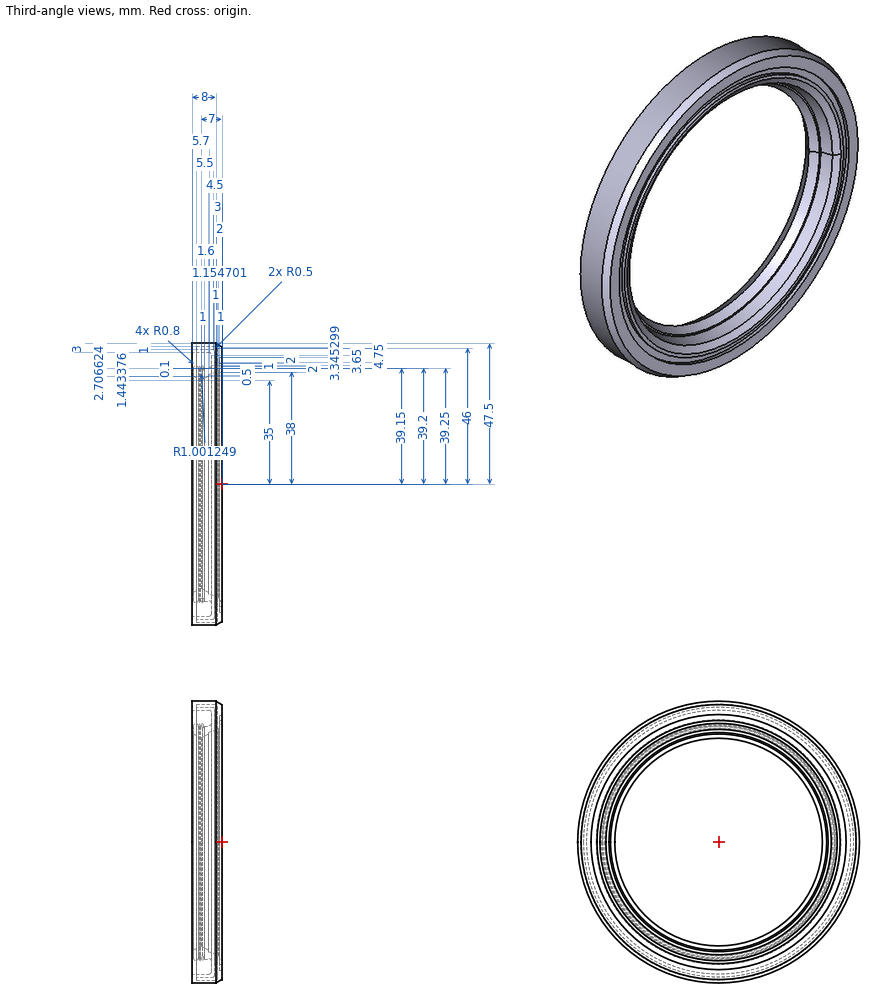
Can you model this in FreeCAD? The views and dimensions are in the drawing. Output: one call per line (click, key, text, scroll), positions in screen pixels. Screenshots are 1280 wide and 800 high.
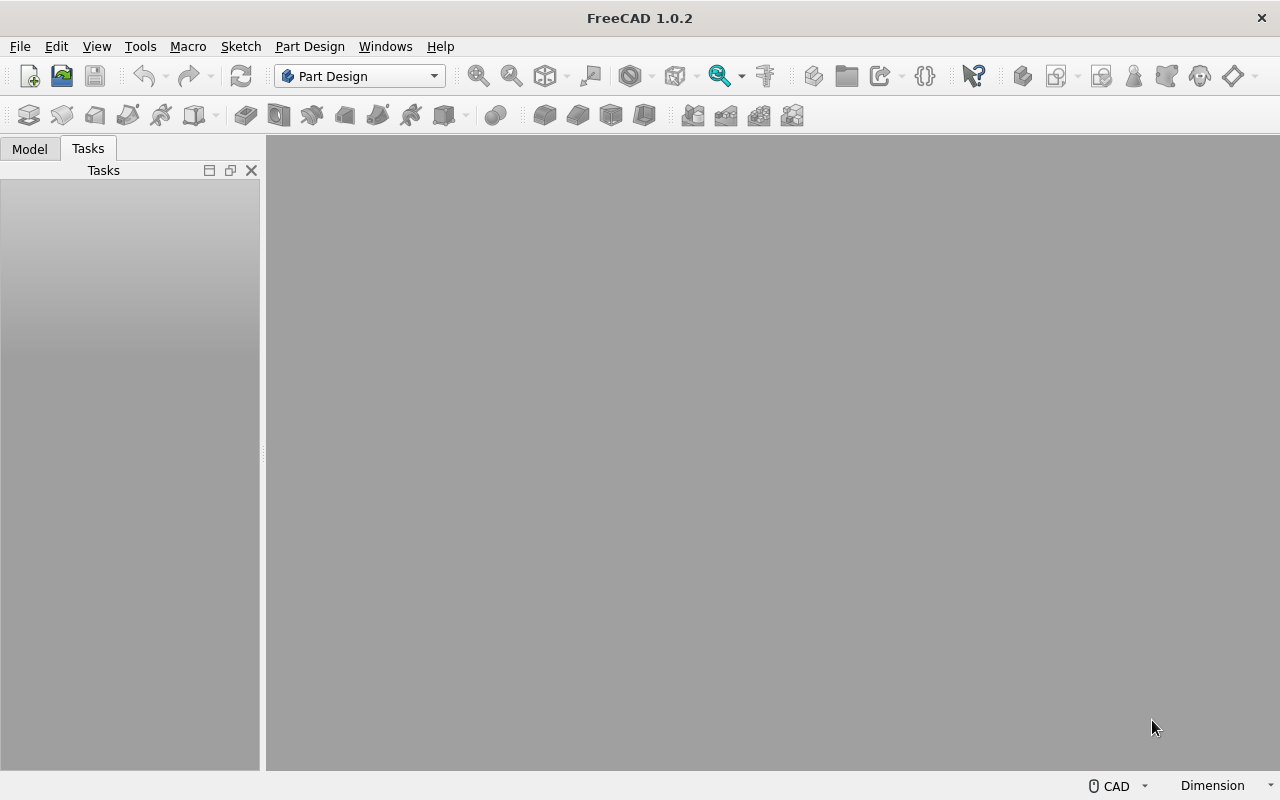
click(29, 76)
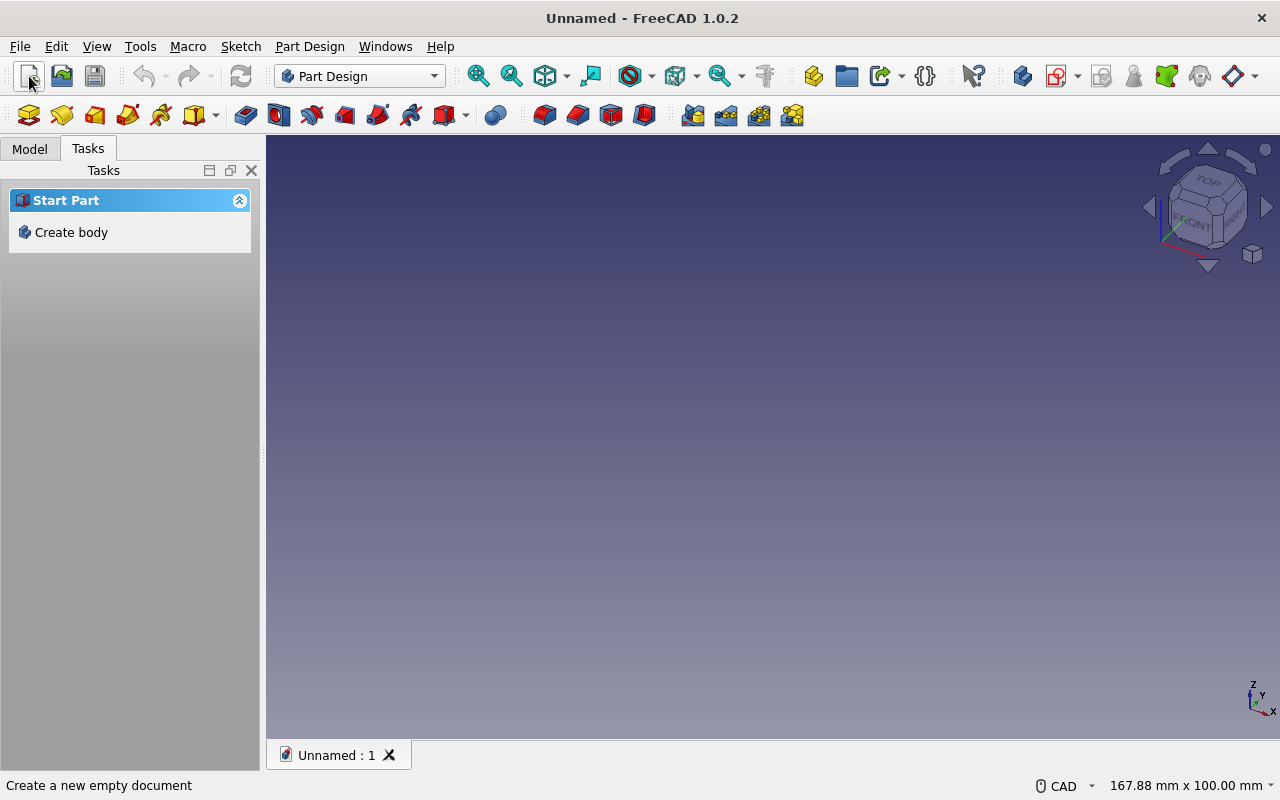
click(1023, 76)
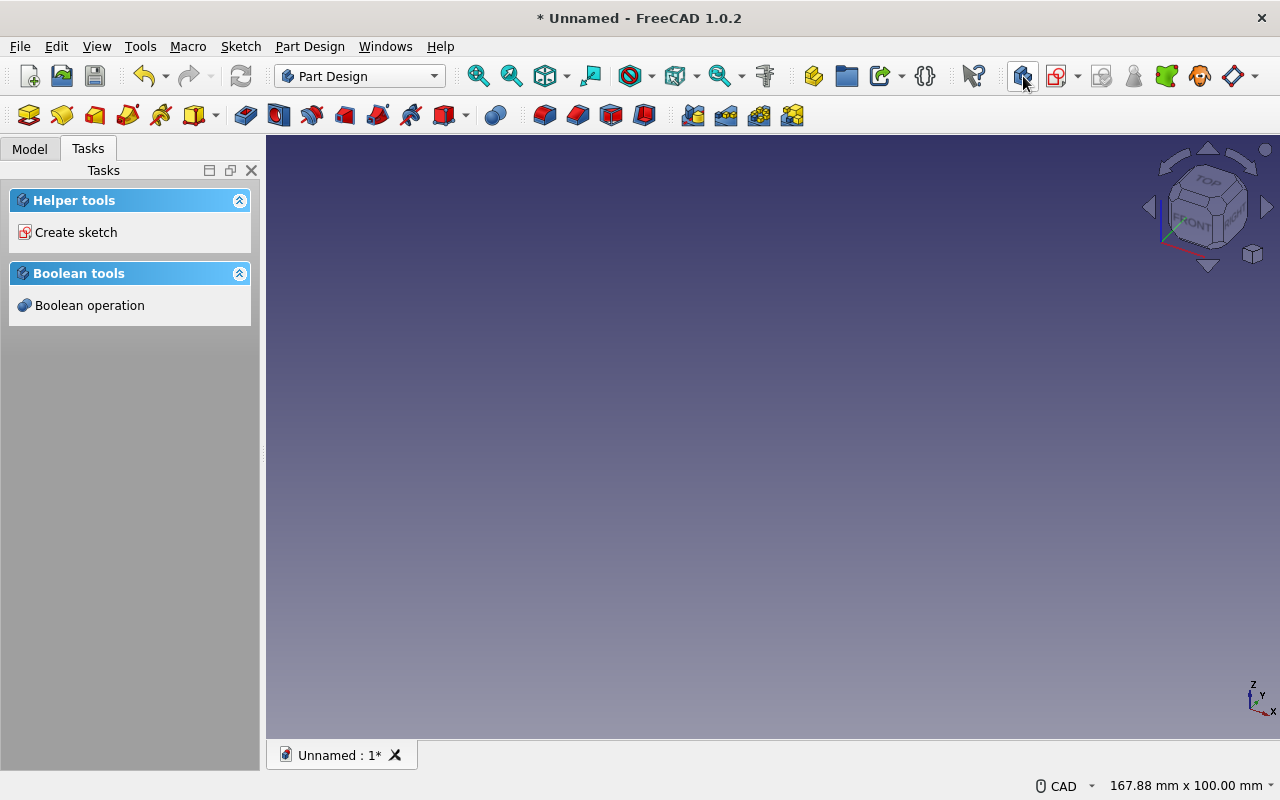
click(30, 148)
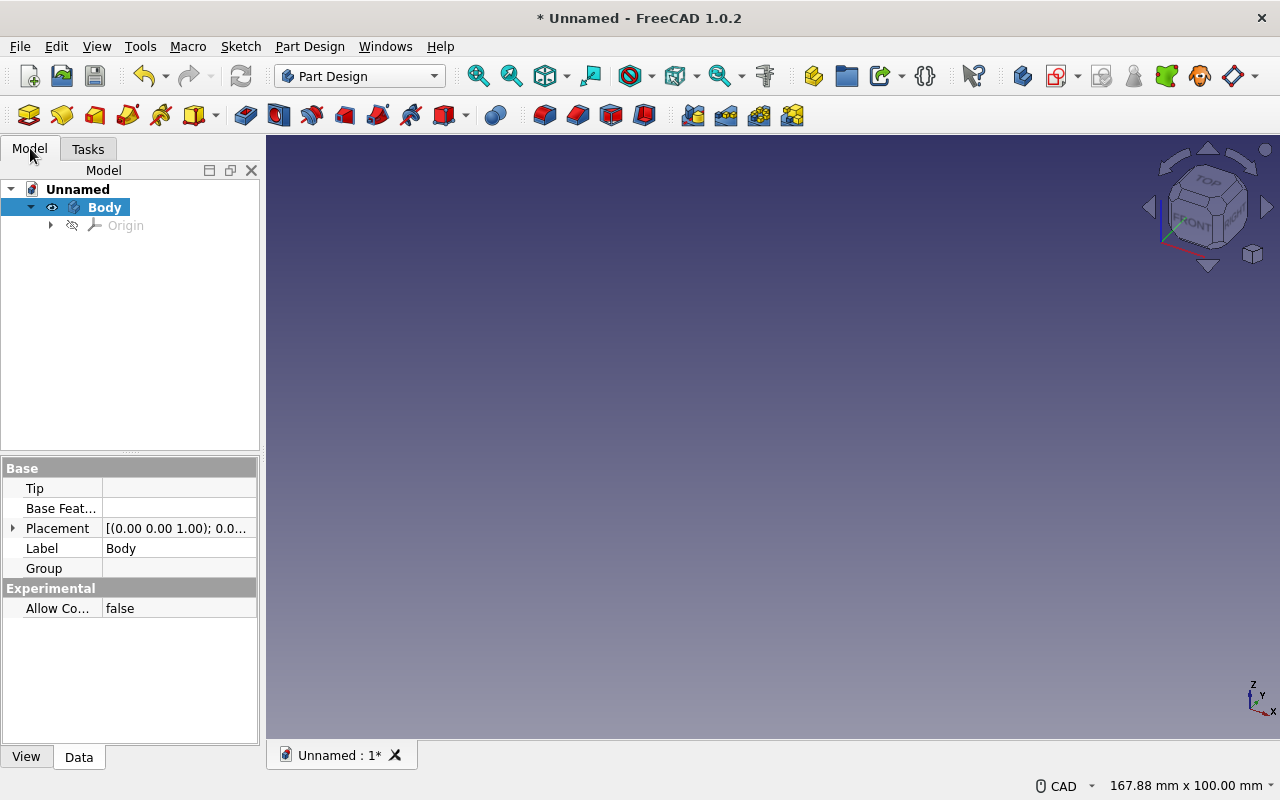
click(97, 207)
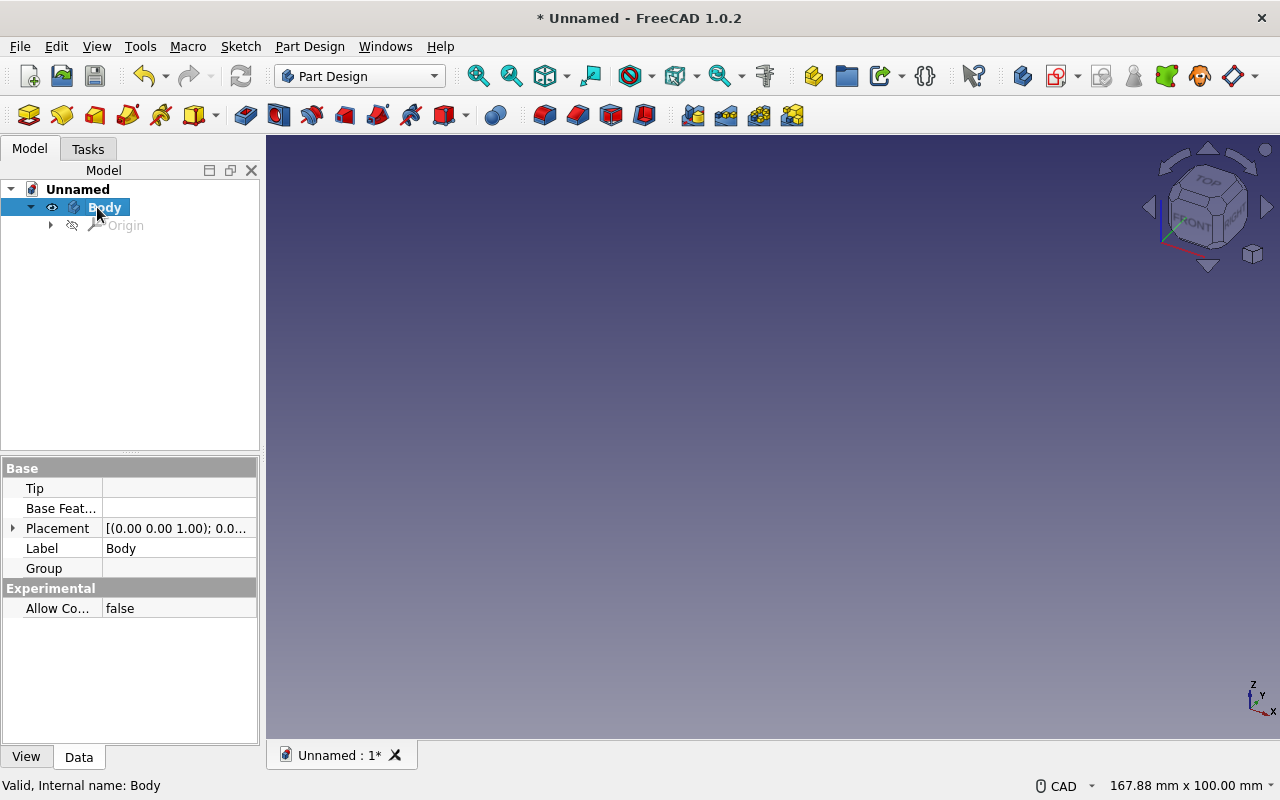
click(148, 608)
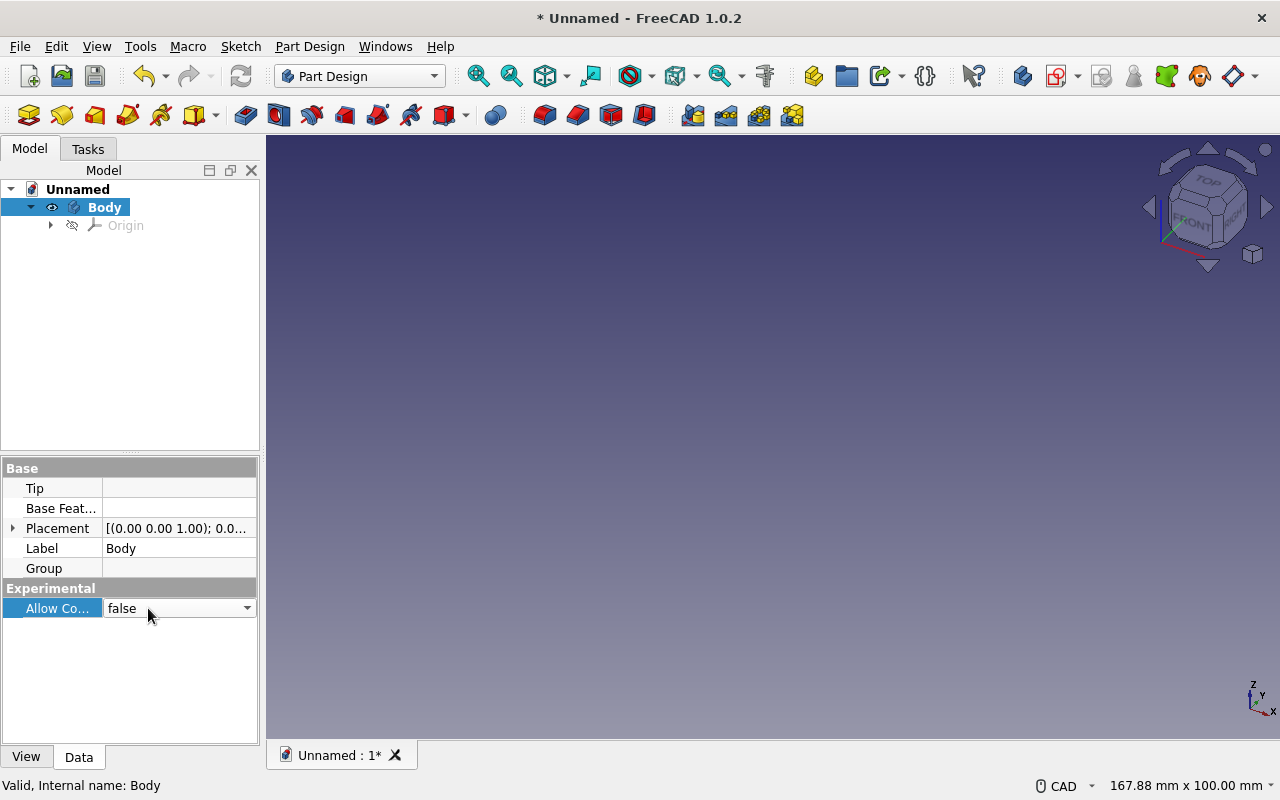
click(148, 608)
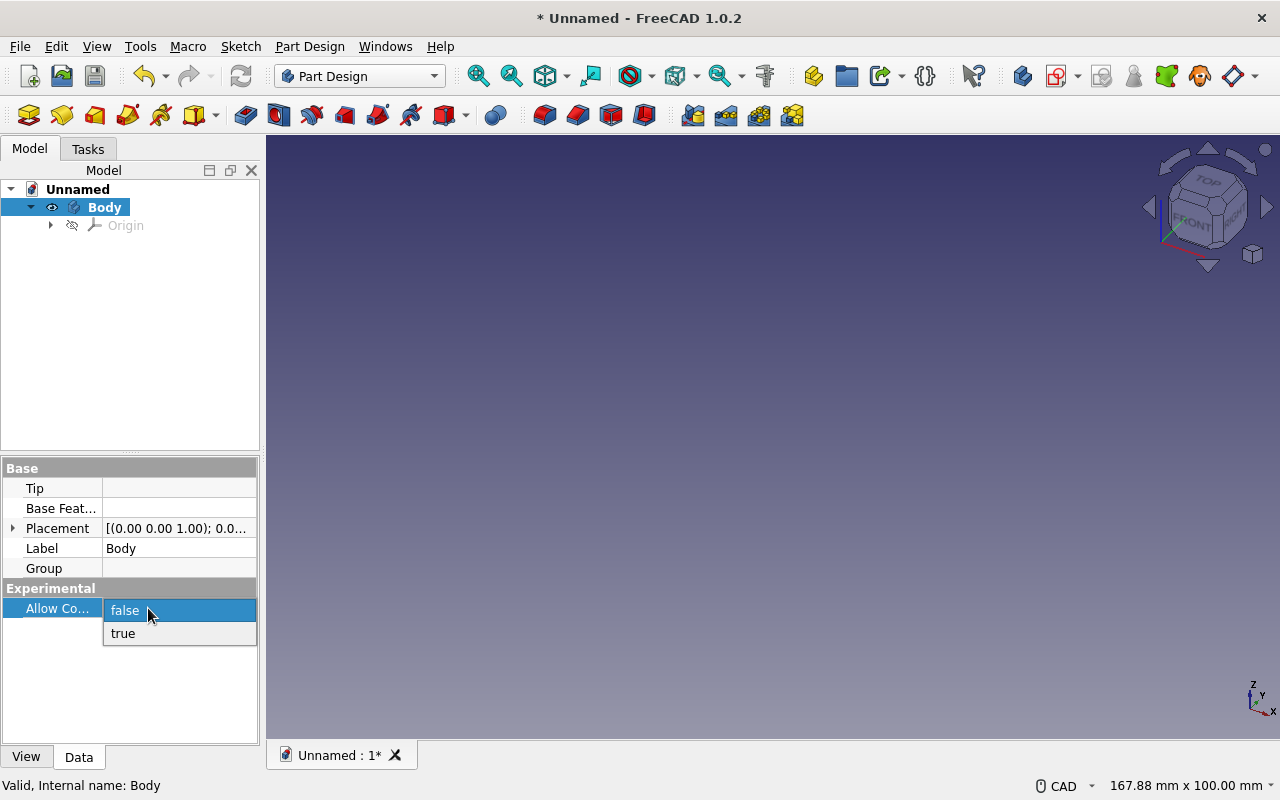
click(178, 634)
key(Return)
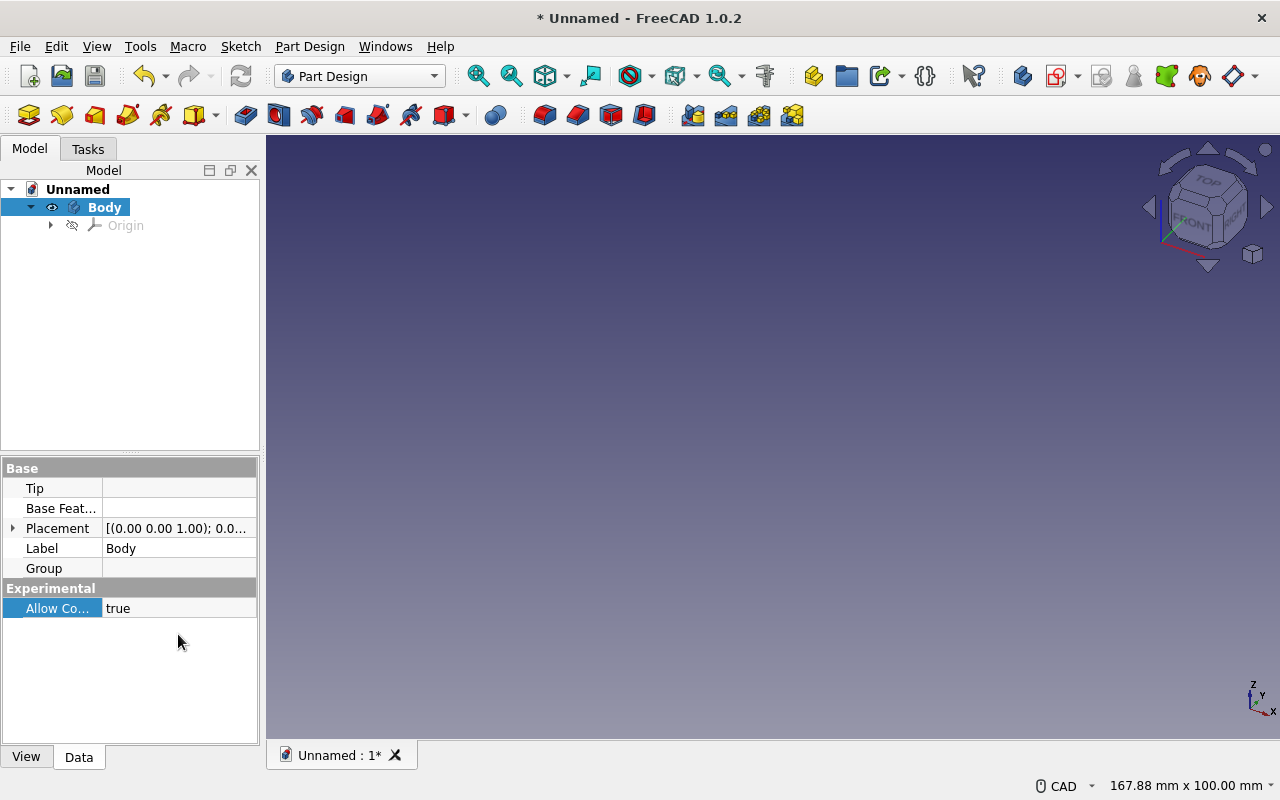
click(306, 699)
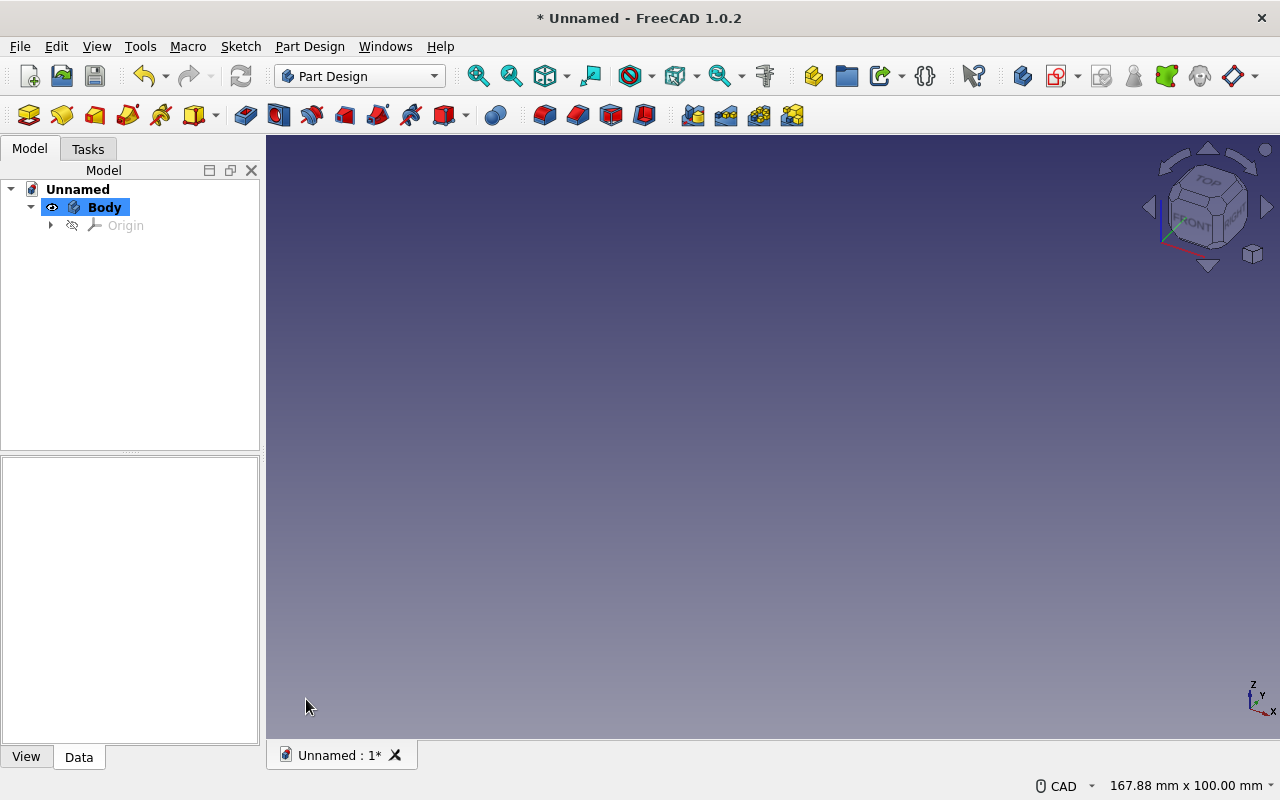
click(1056, 76)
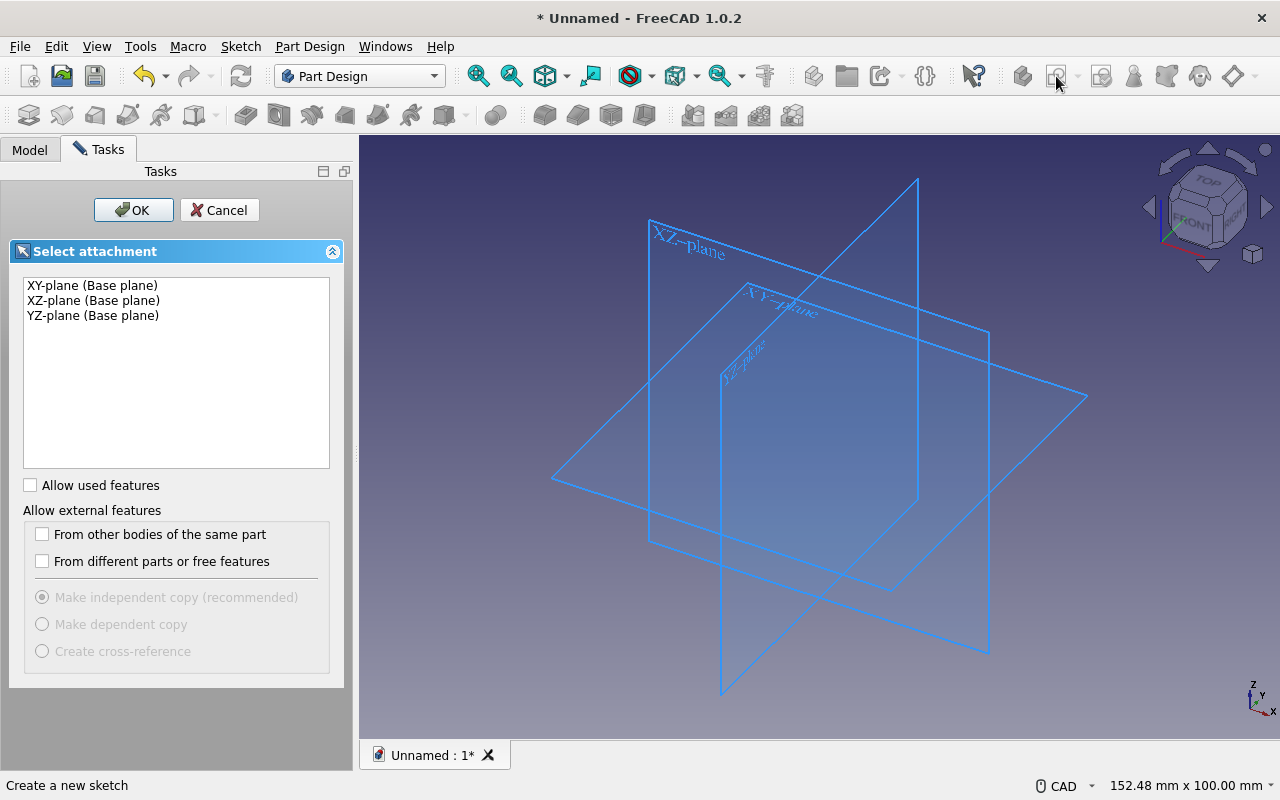
click(84, 286)